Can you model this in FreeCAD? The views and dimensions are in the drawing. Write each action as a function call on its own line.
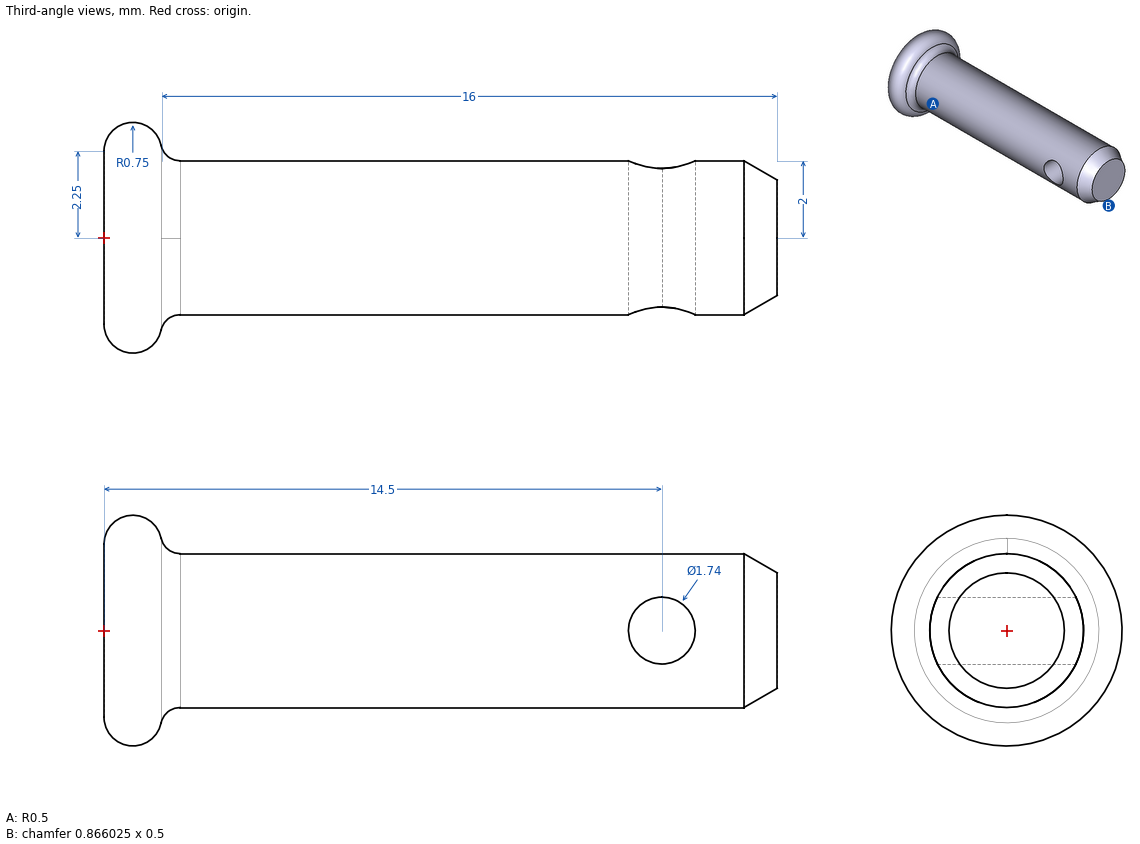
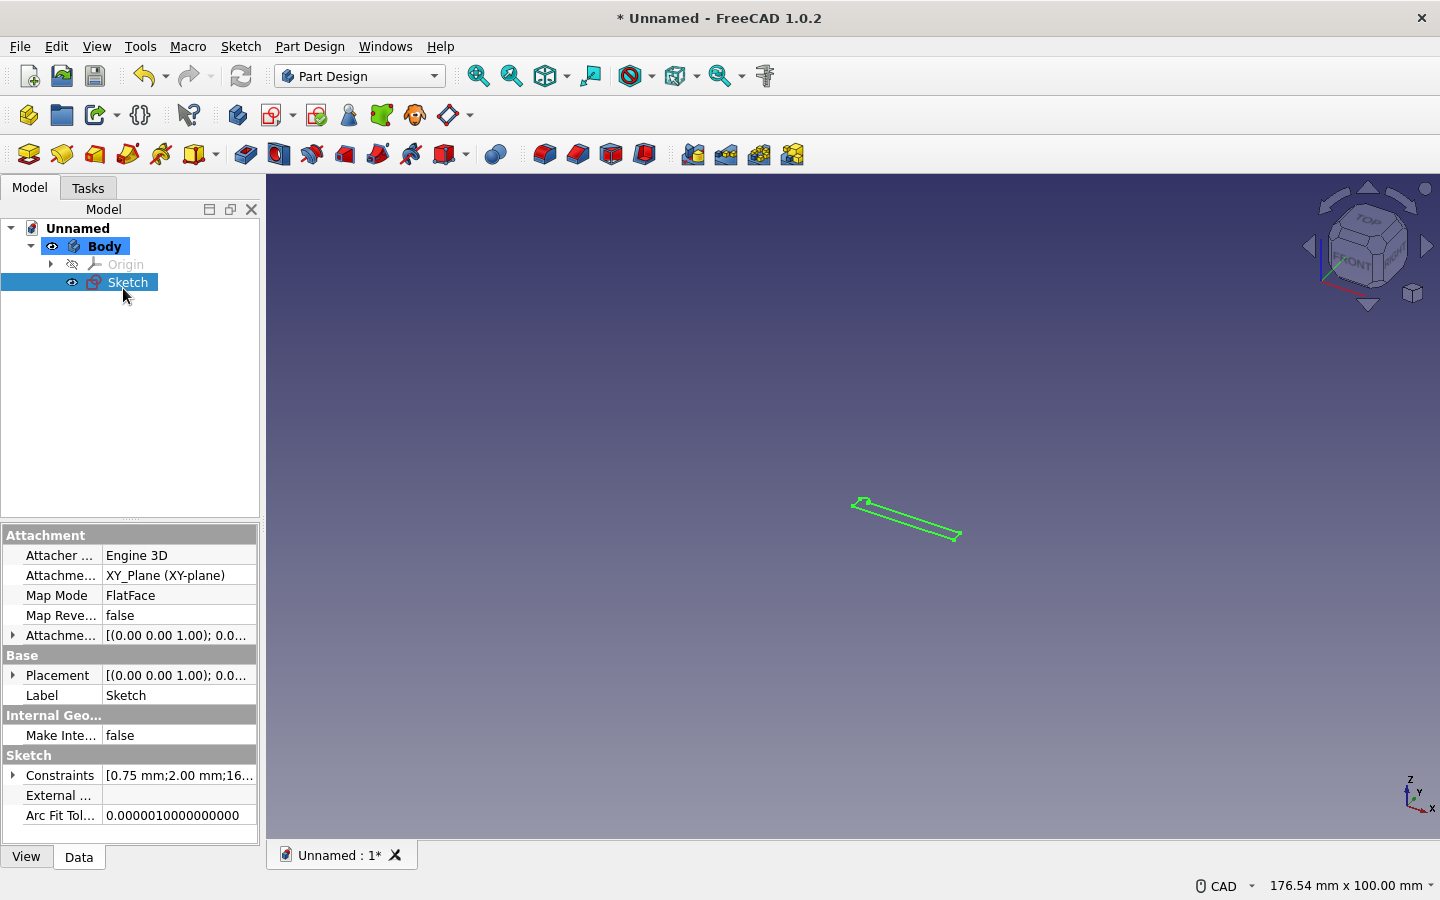
click(62, 154)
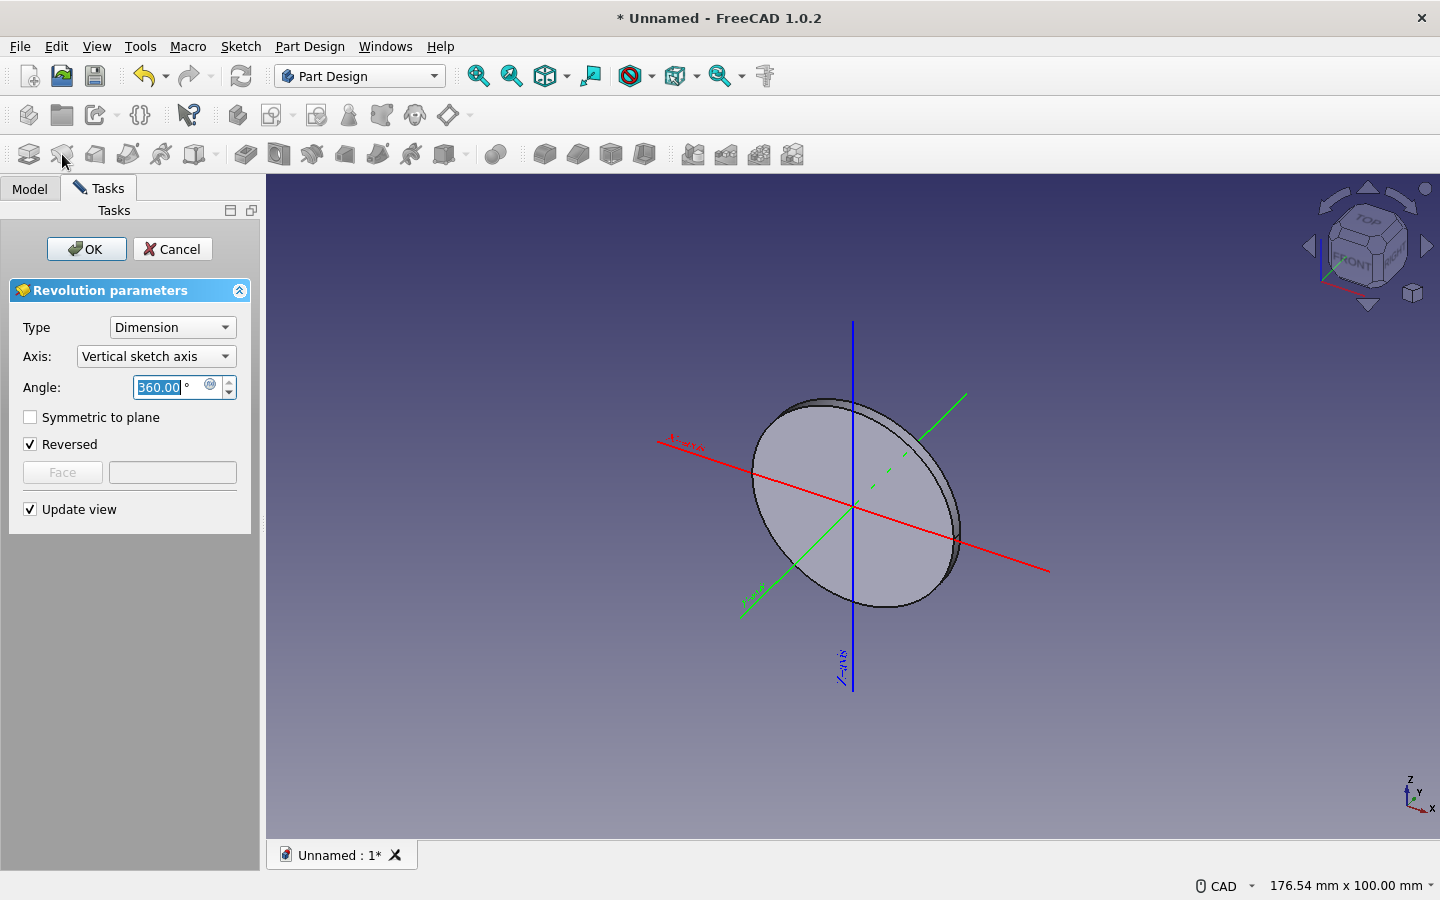
click(157, 356)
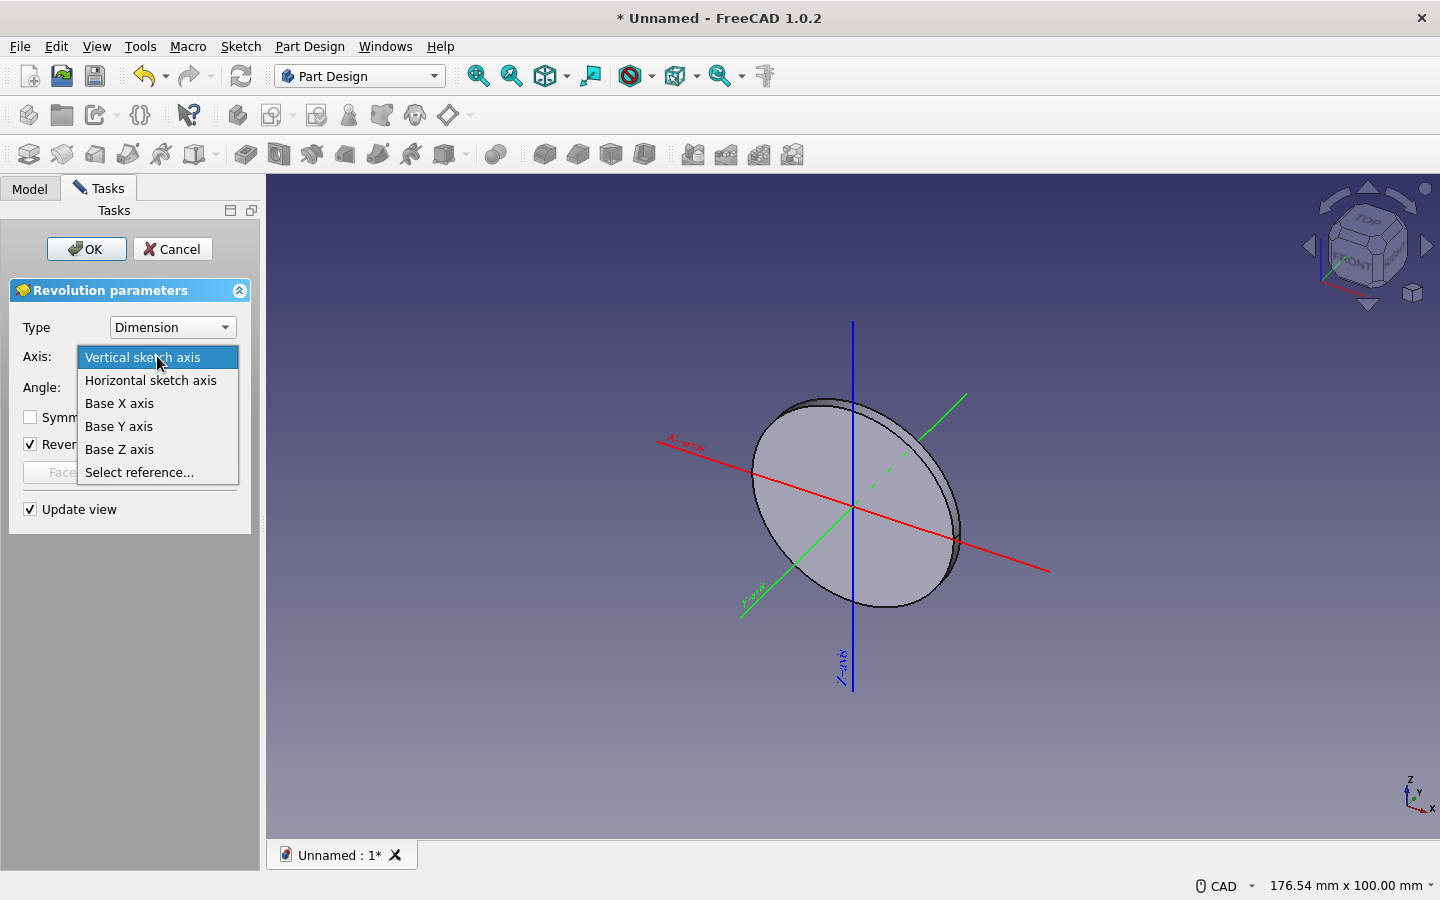
click(156, 380)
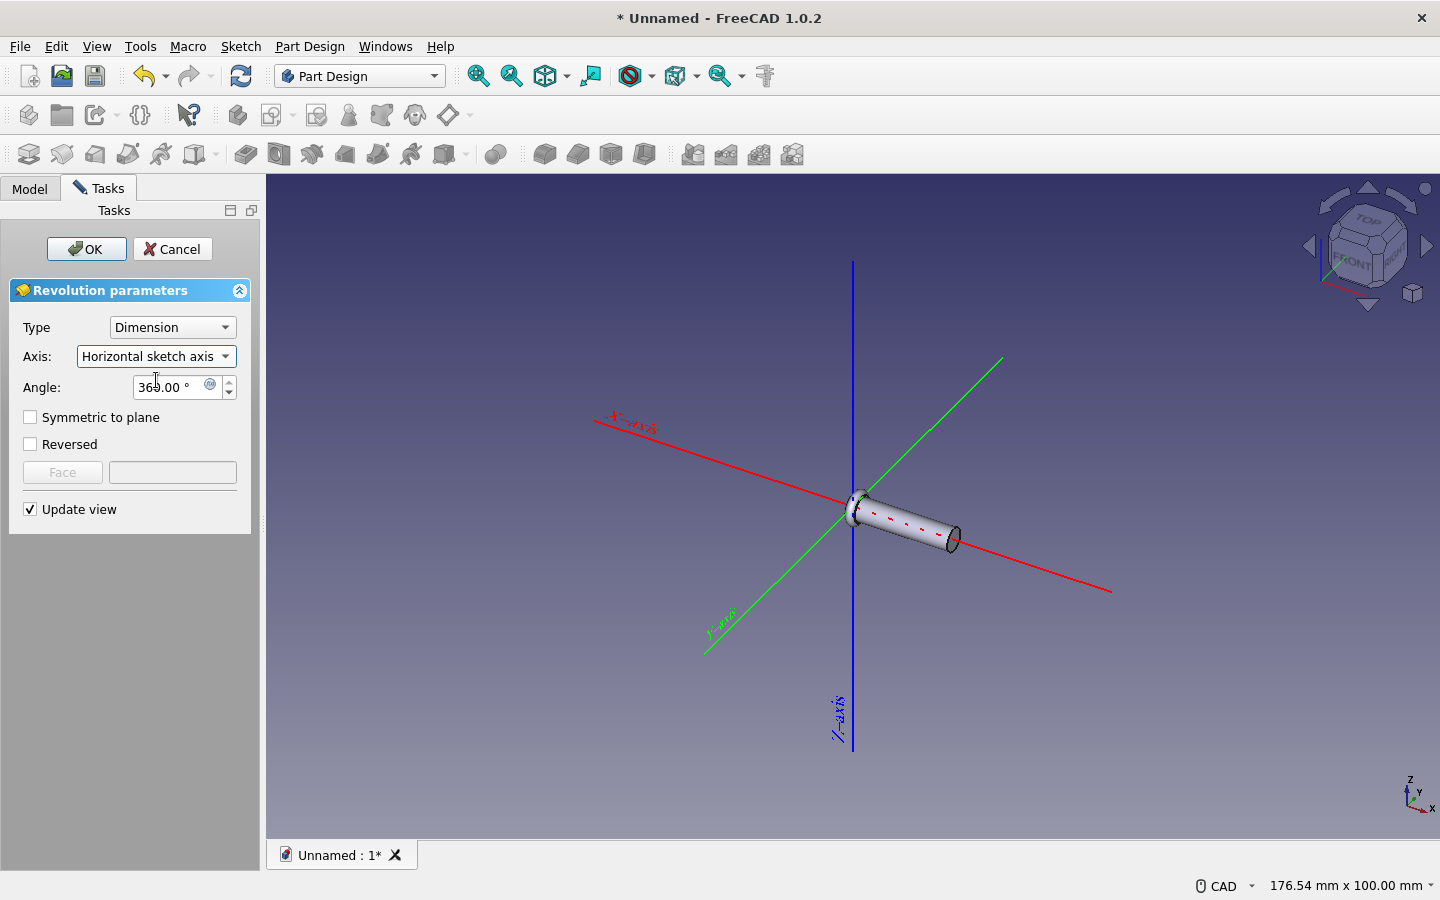
click(87, 249)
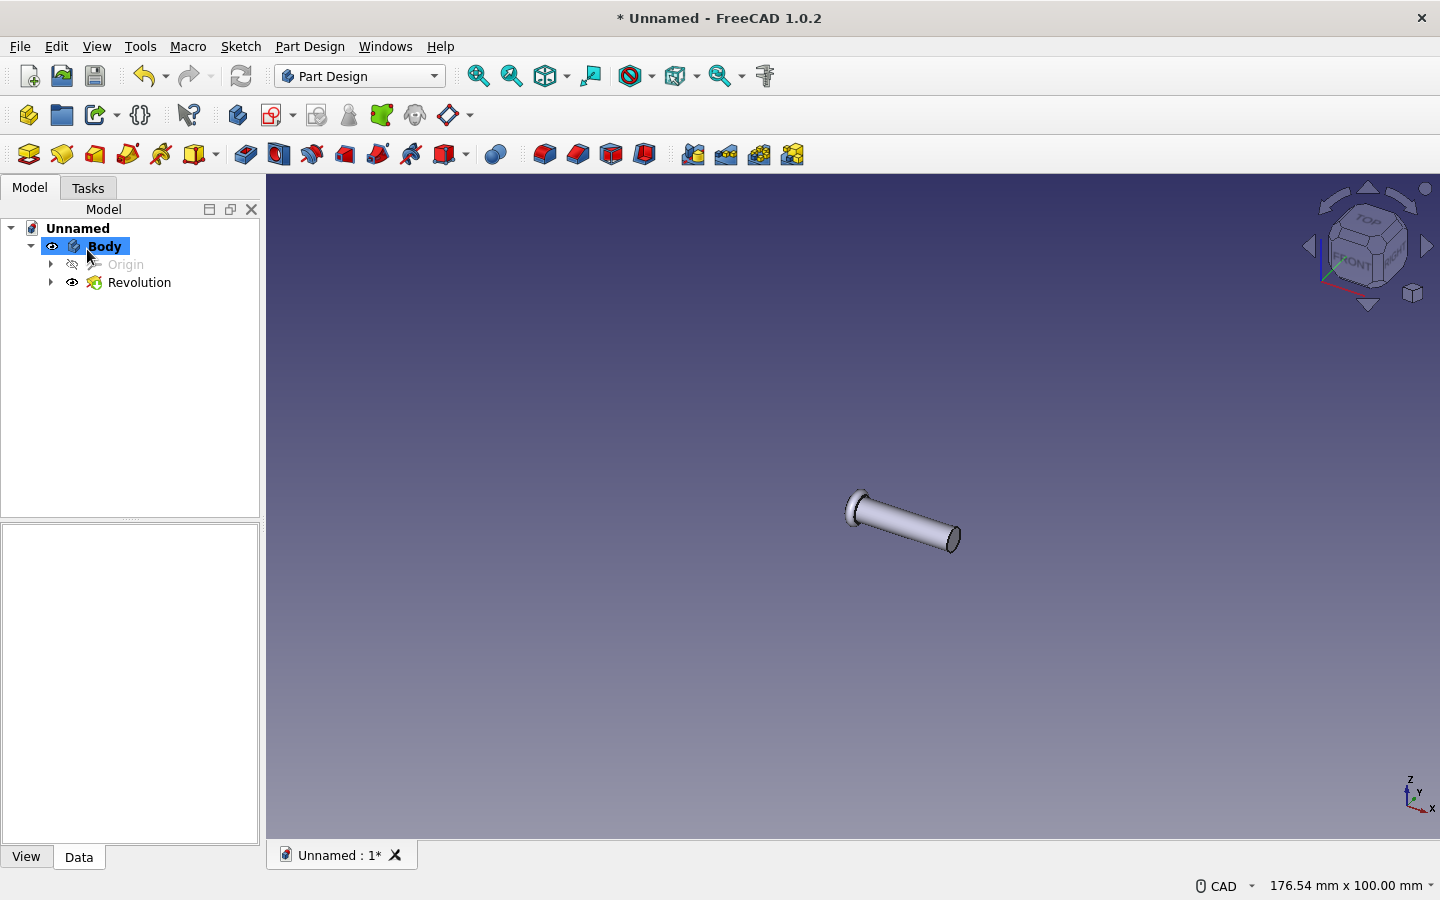
click(479, 76)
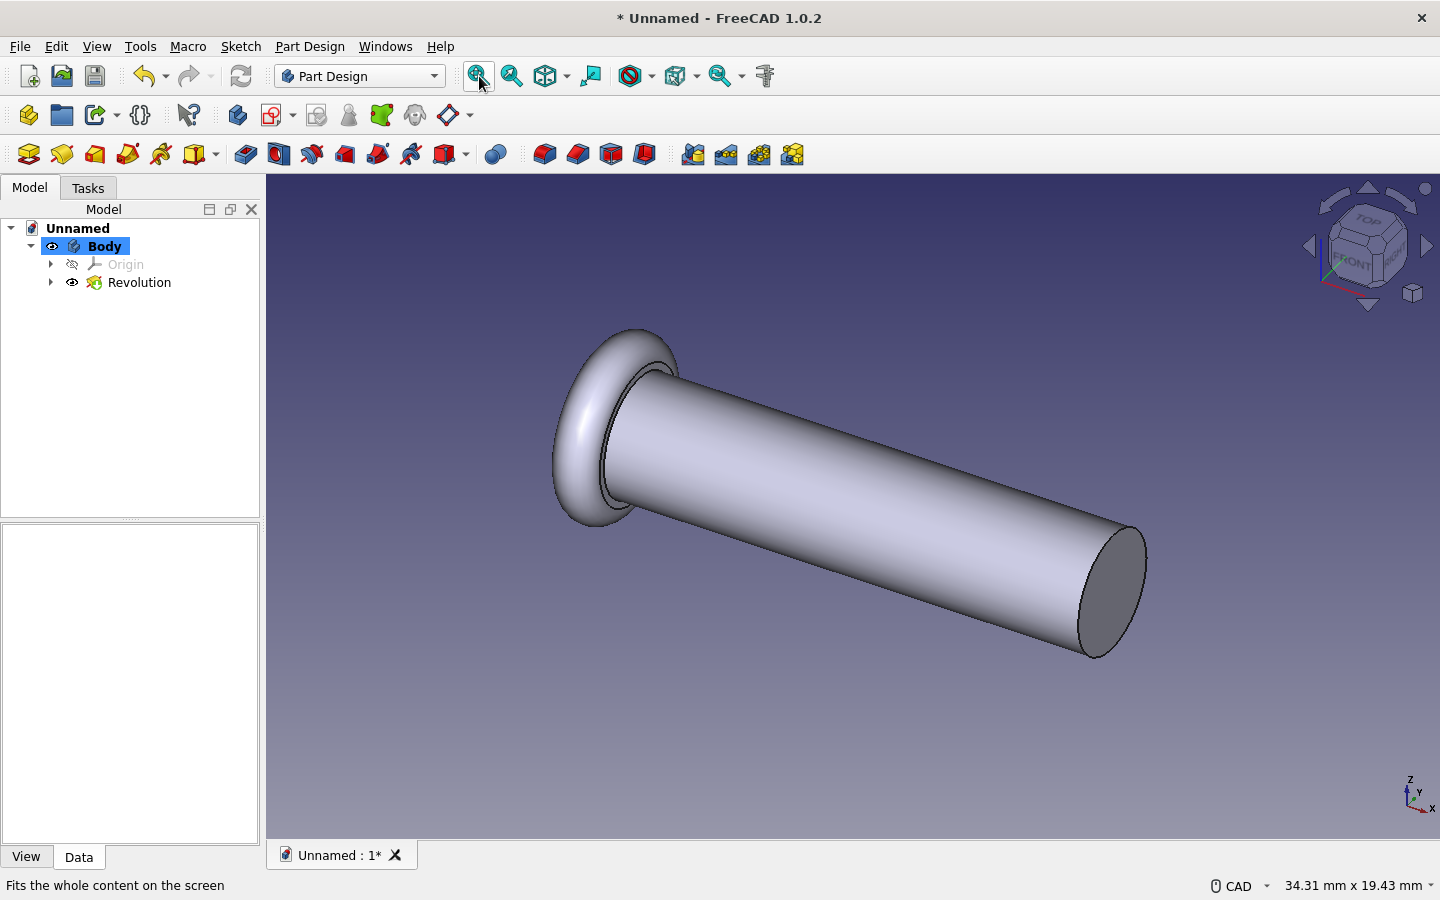
key(0)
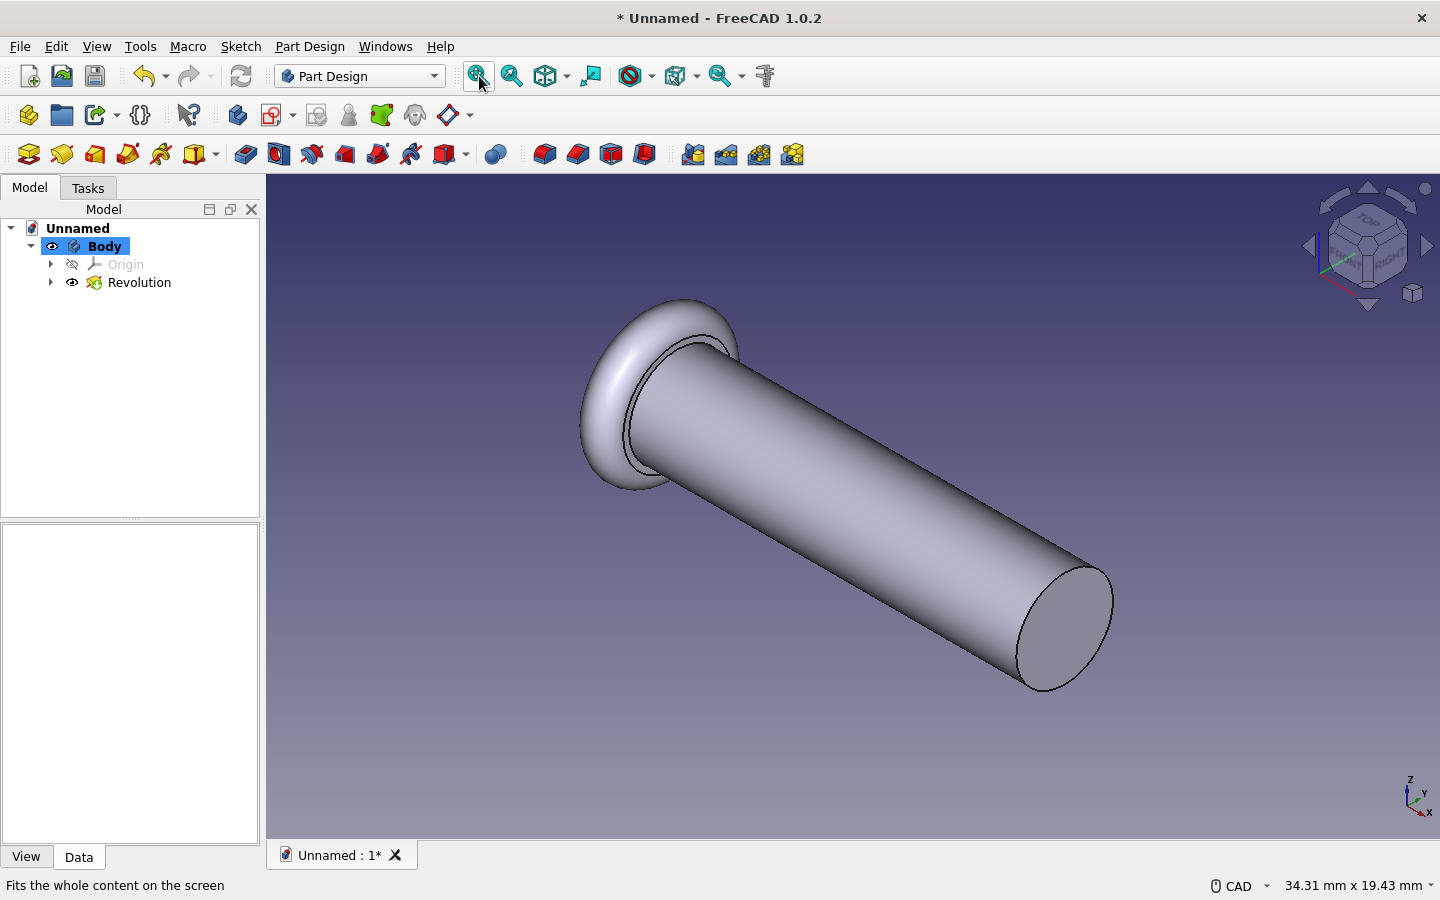
key(2)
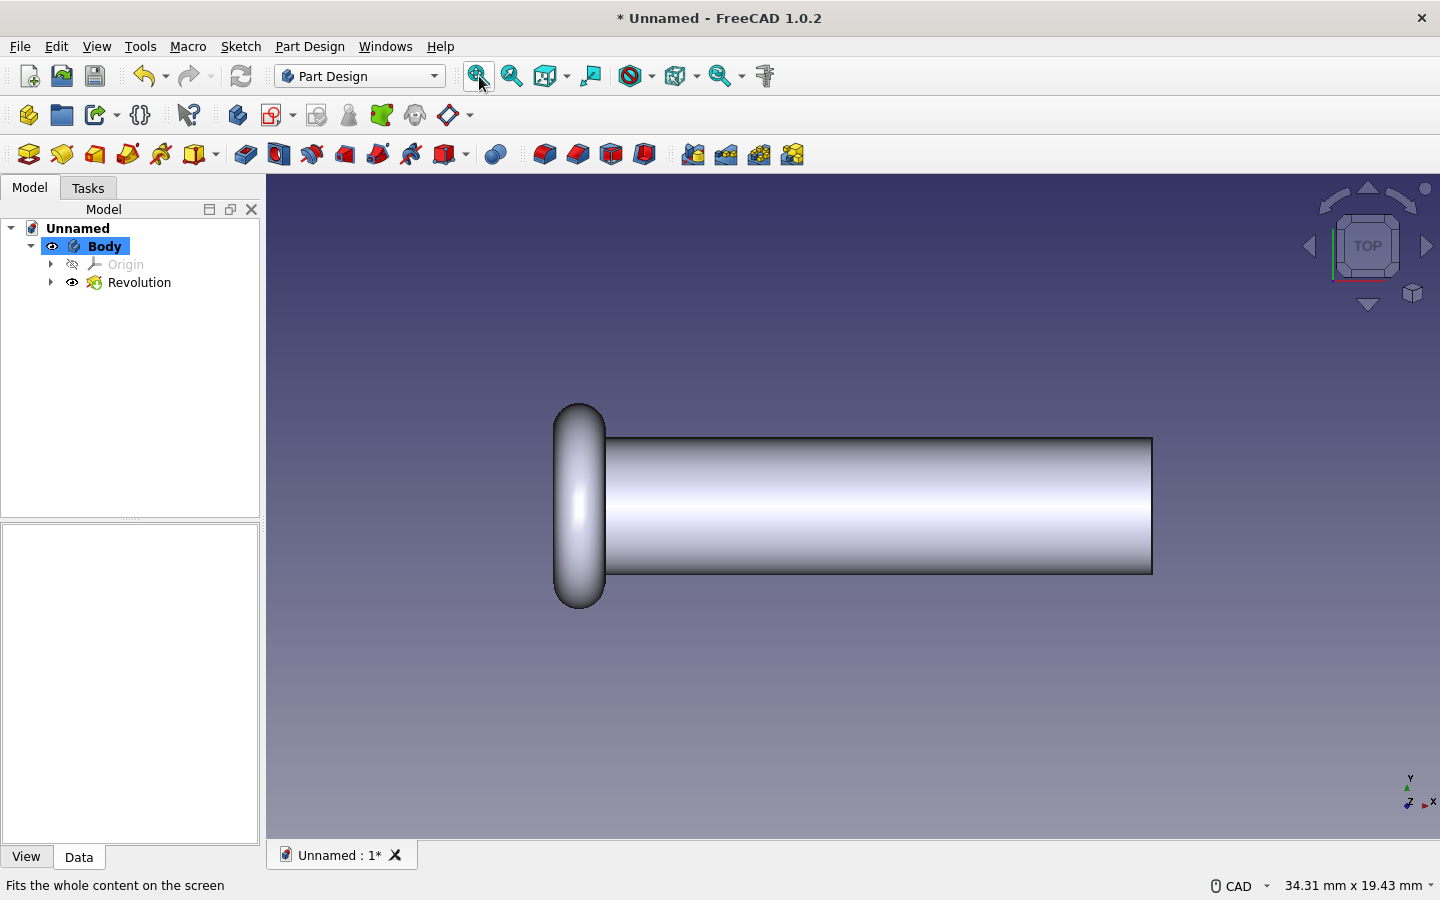
key(1)